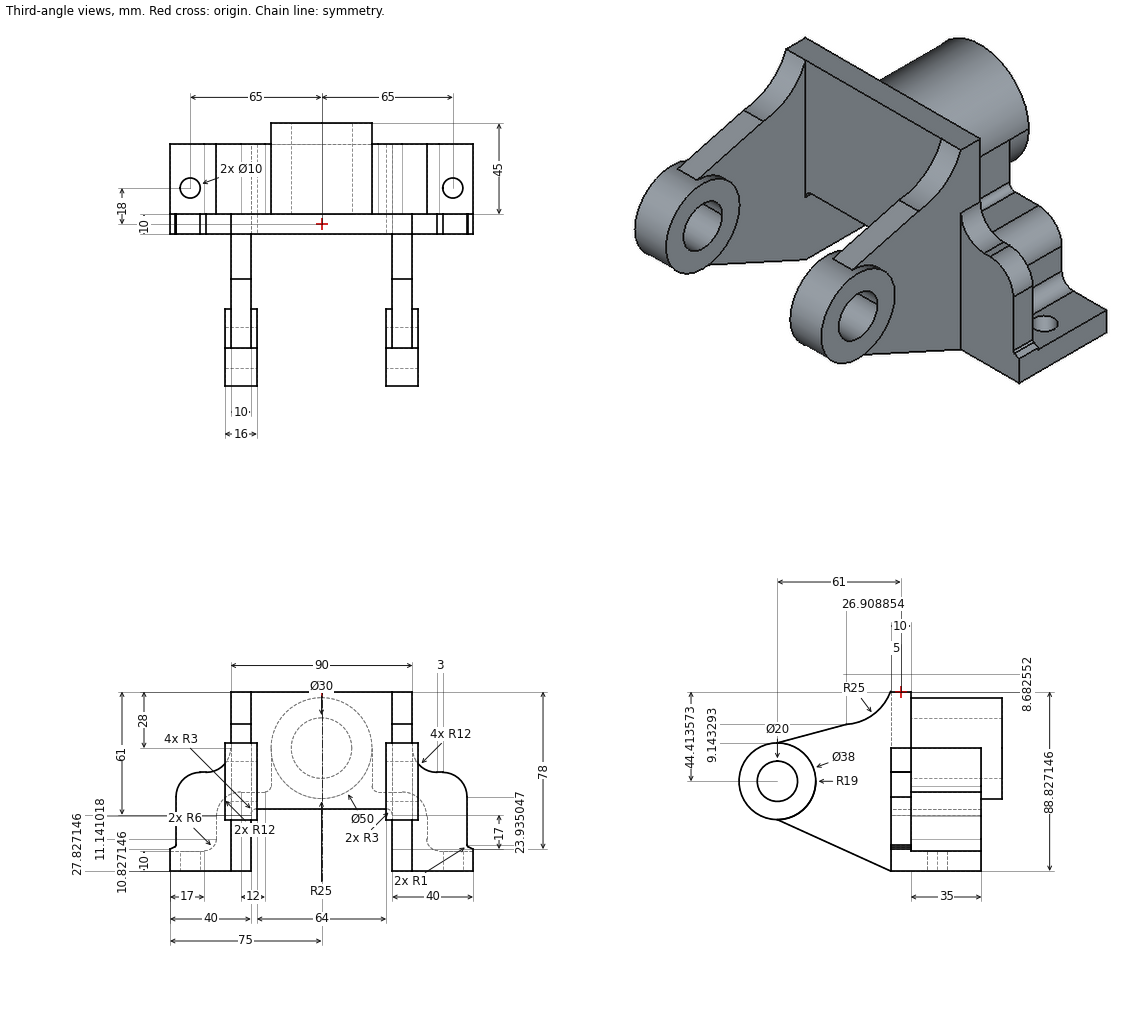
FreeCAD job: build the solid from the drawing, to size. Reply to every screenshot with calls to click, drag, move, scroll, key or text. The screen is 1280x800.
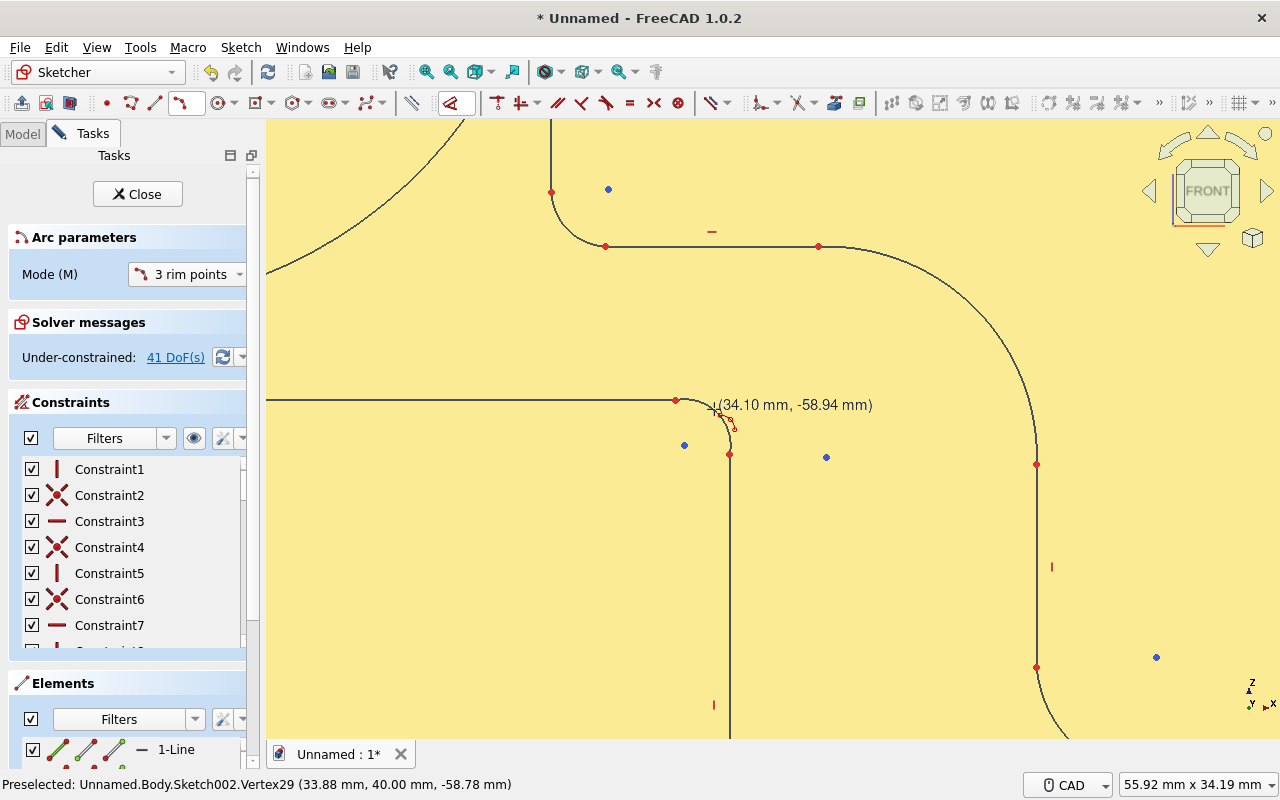
scroll(858, 500, down, 8)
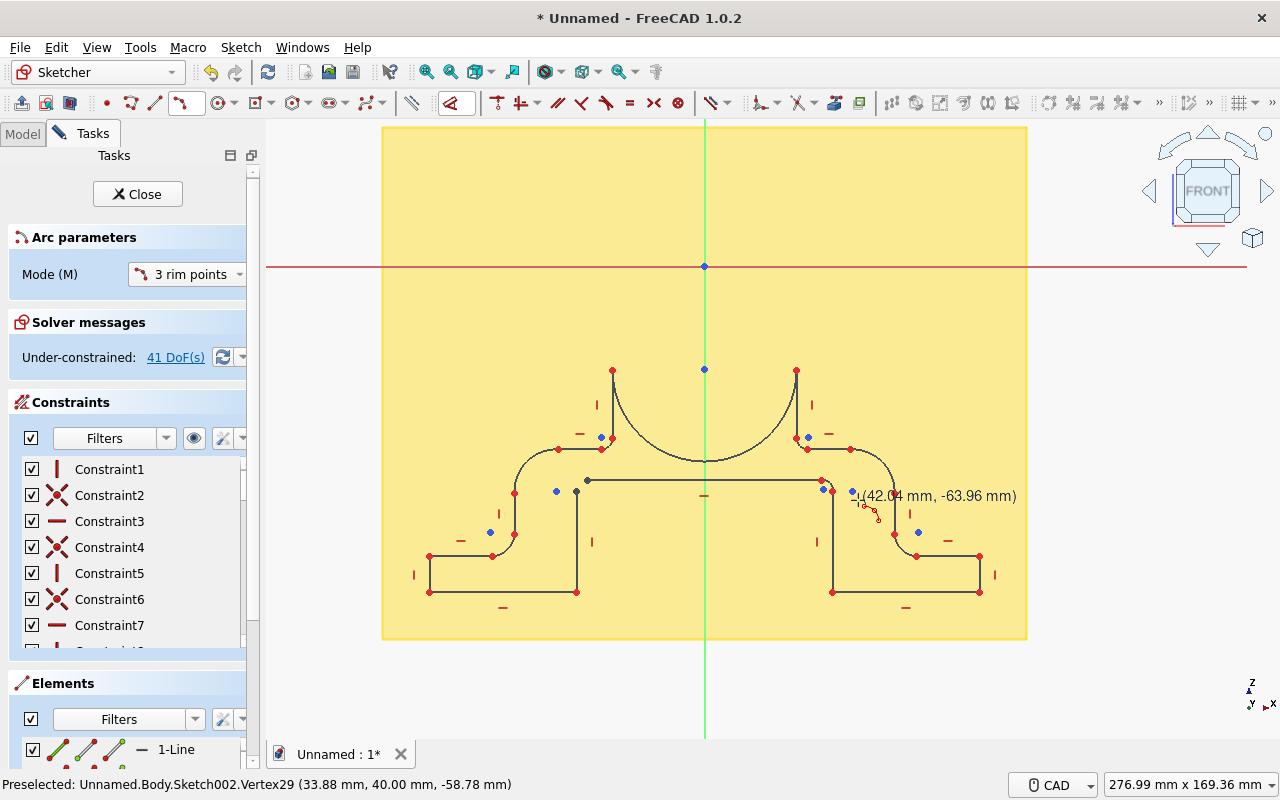
click(588, 480)
click(577, 491)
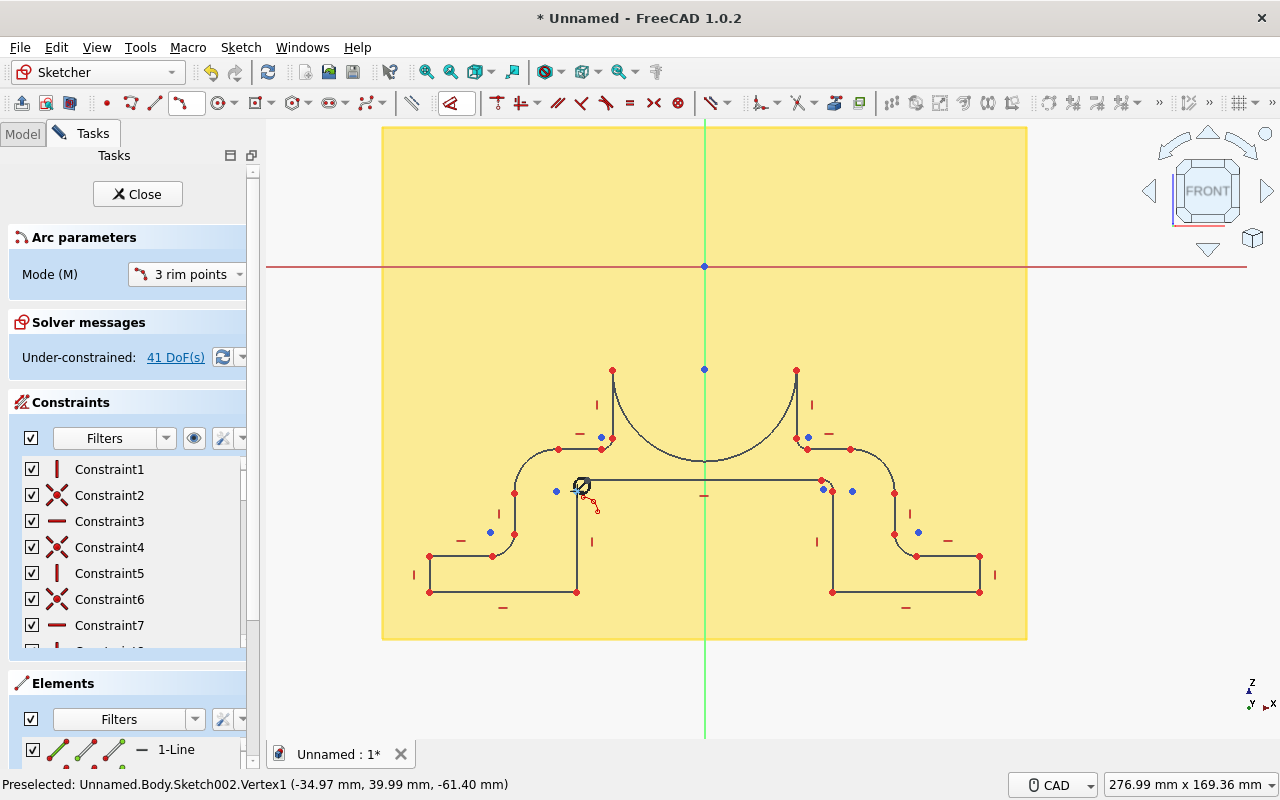
scroll(580, 482, up, 8)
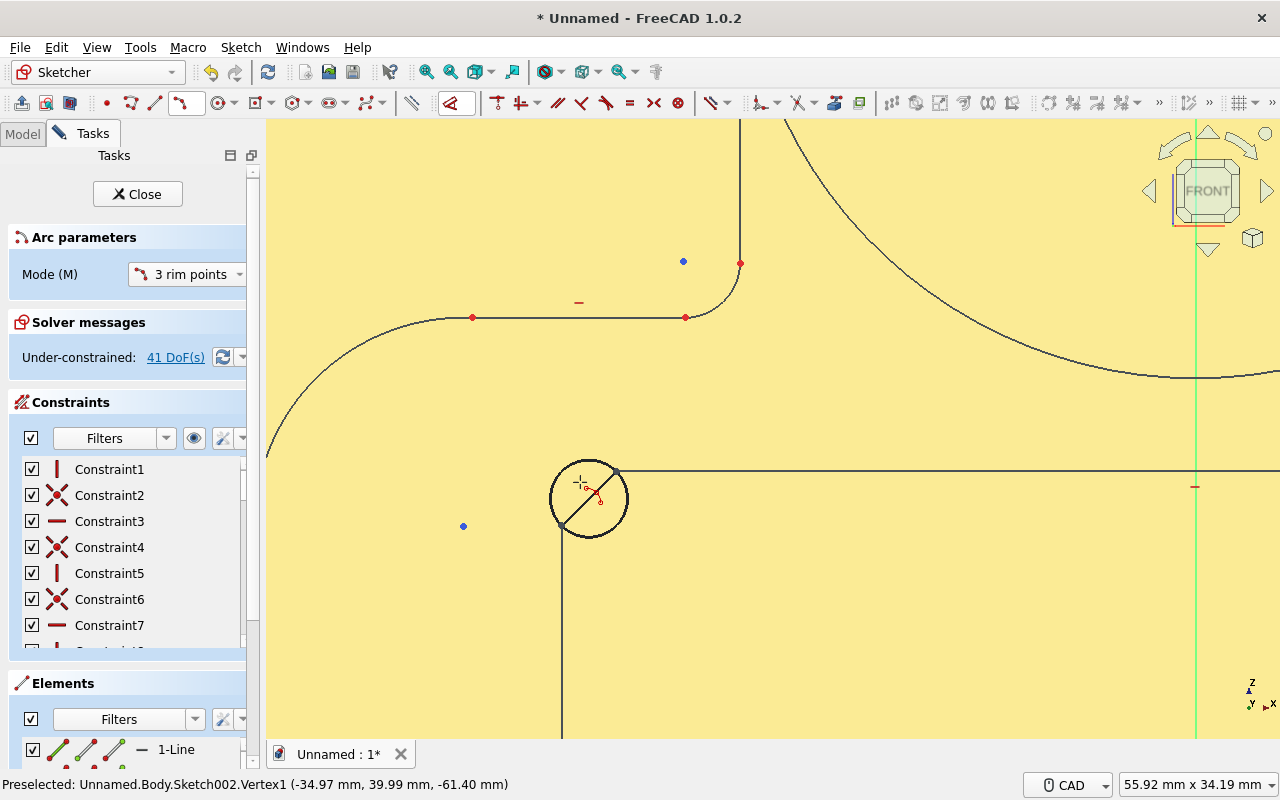
click(577, 480)
key(Escape)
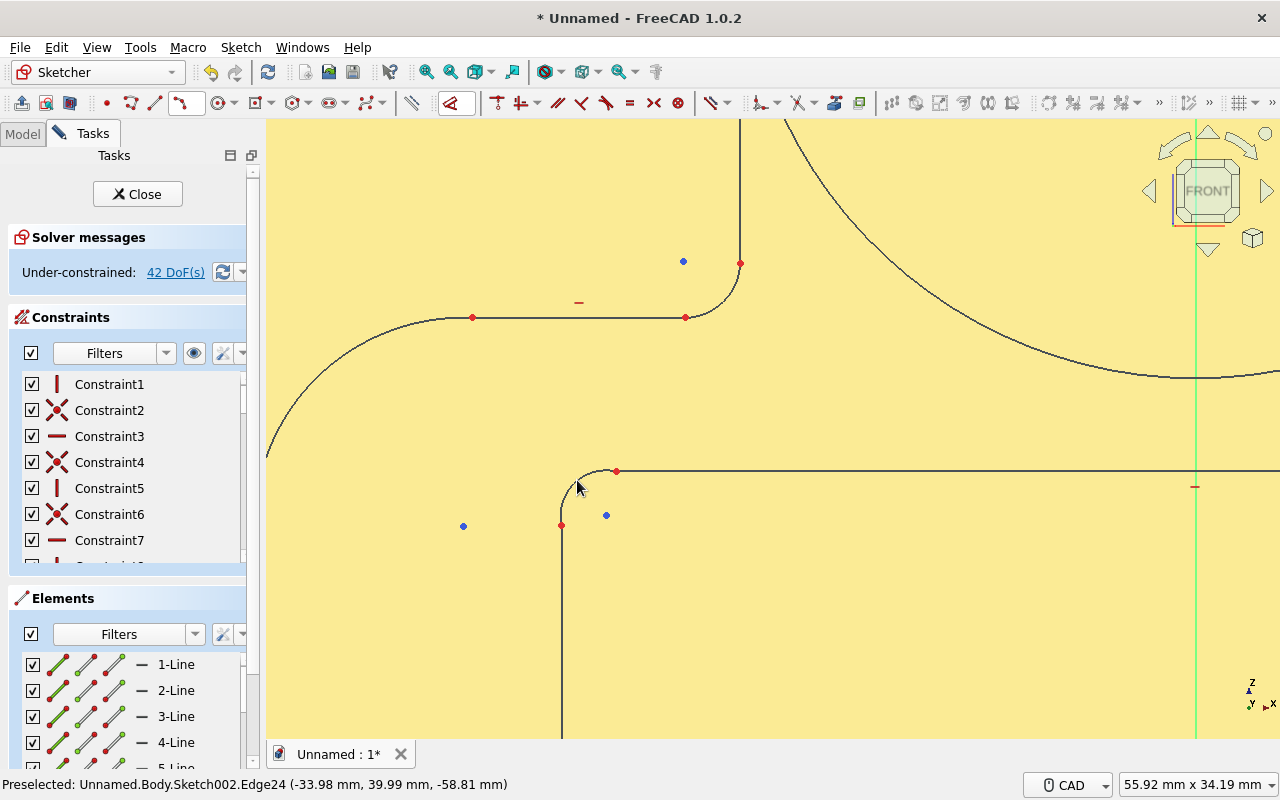
scroll(580, 482, down, 8)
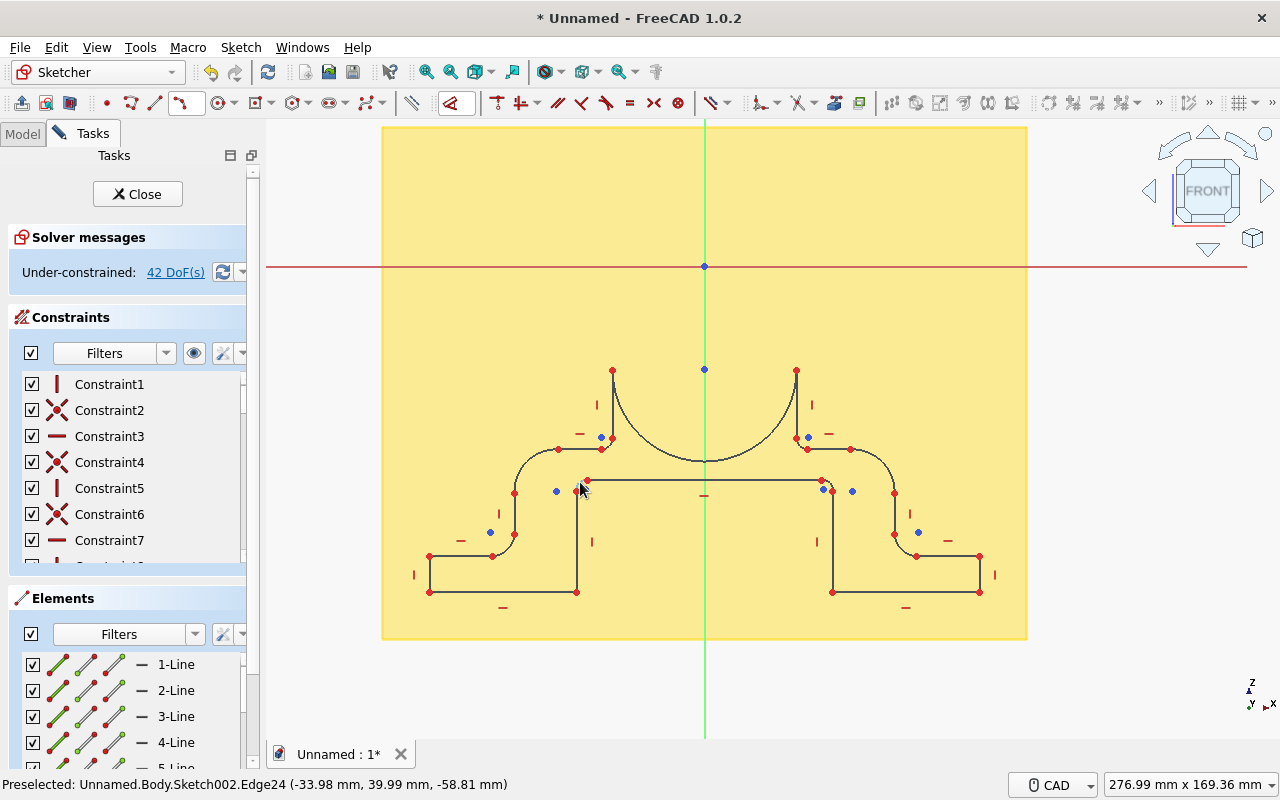
click(577, 522)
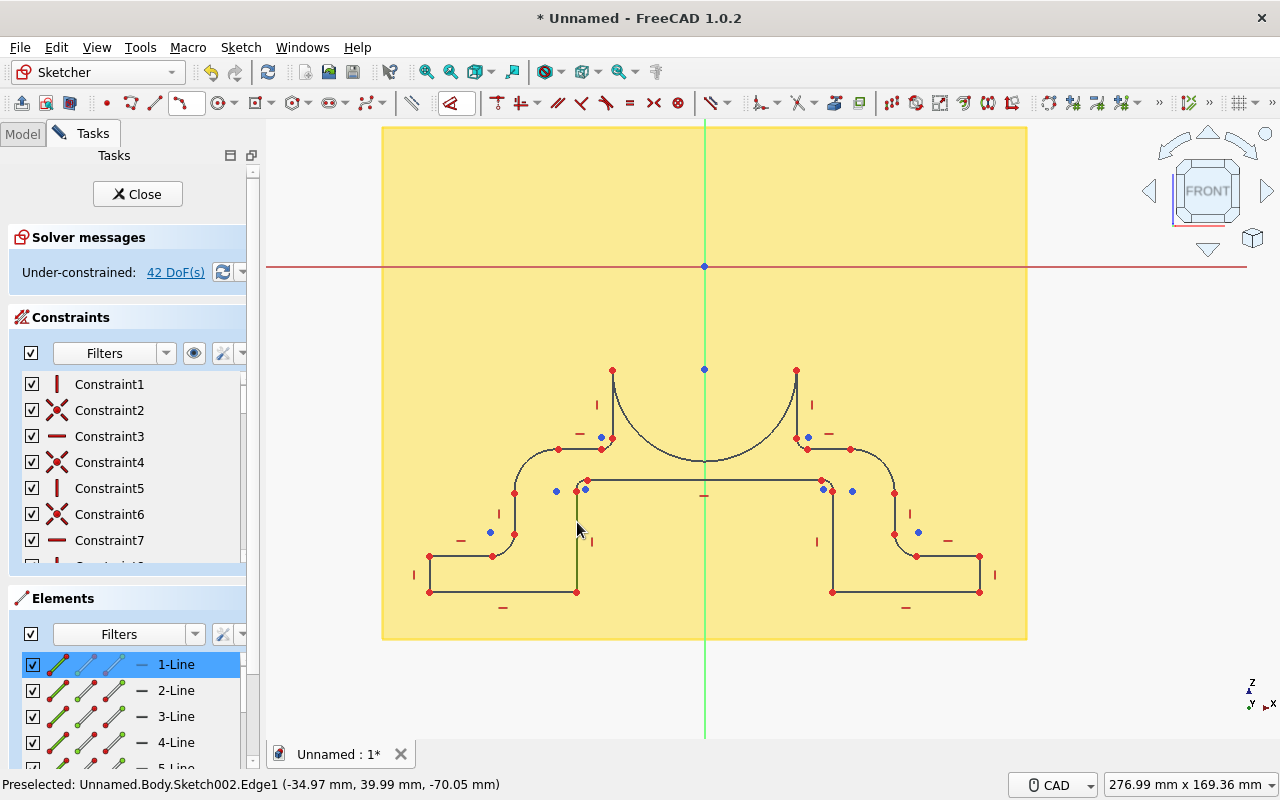
scroll(579, 483, up, 3)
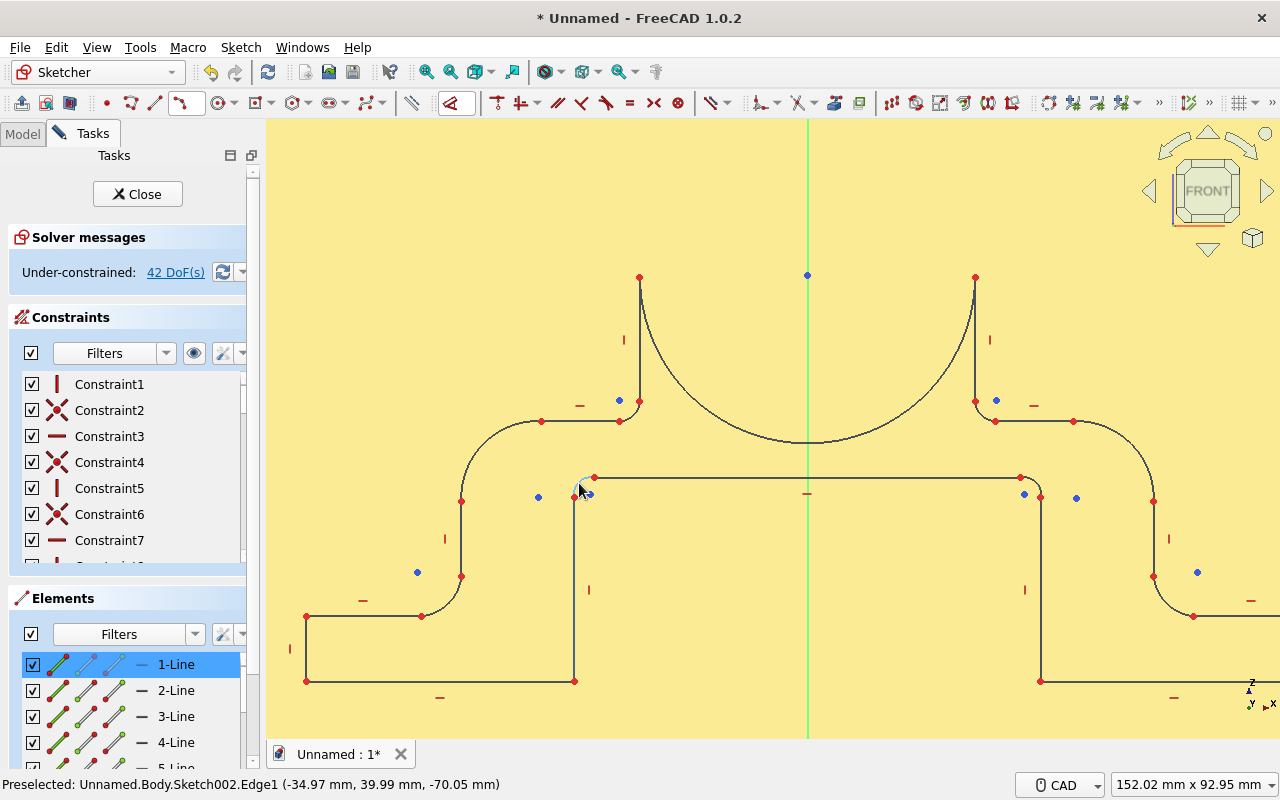
click(579, 482)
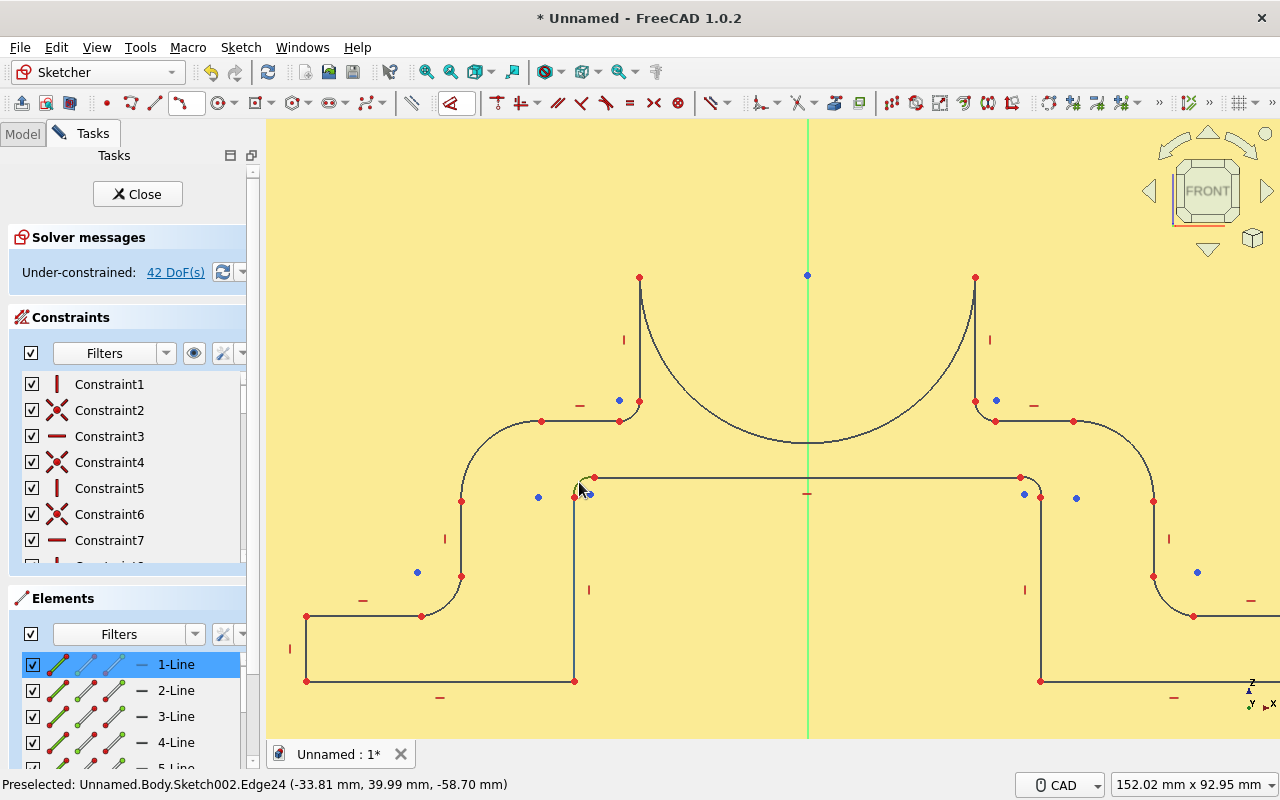
click(606, 104)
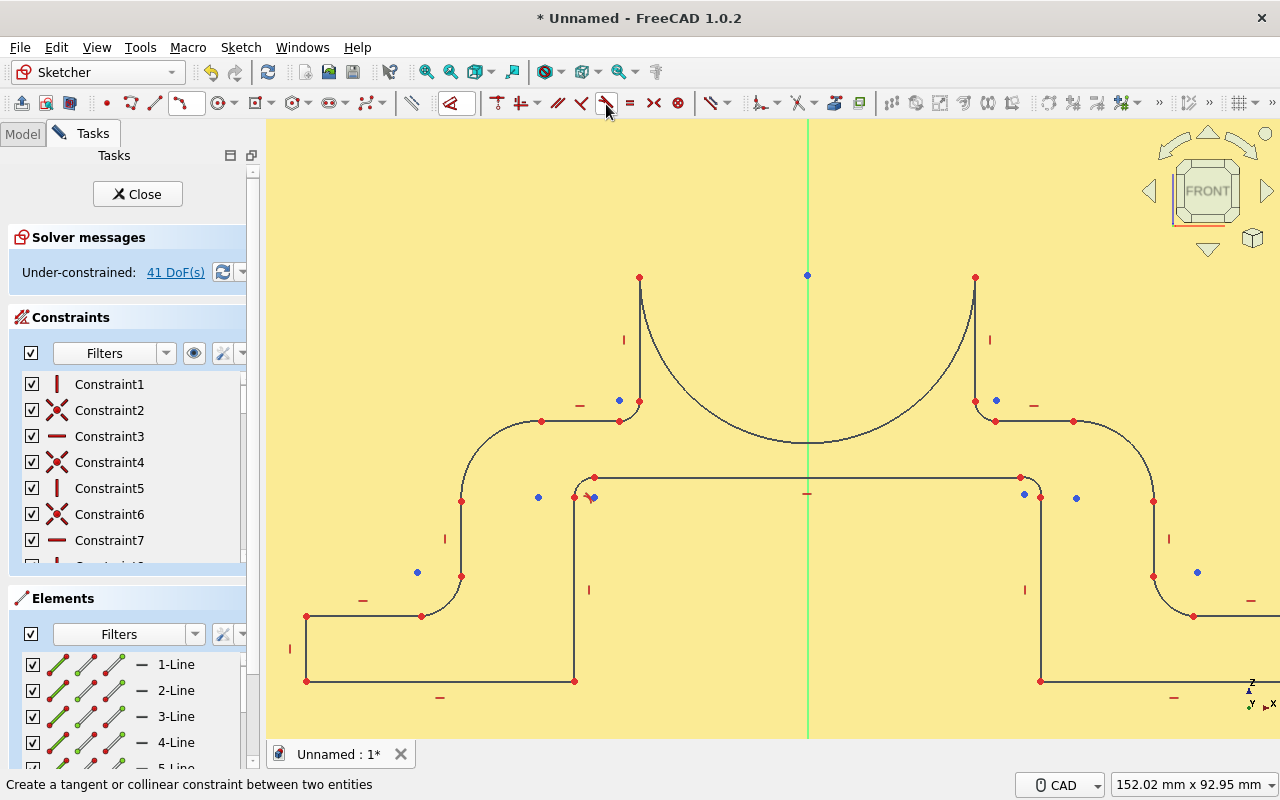
click(341, 616)